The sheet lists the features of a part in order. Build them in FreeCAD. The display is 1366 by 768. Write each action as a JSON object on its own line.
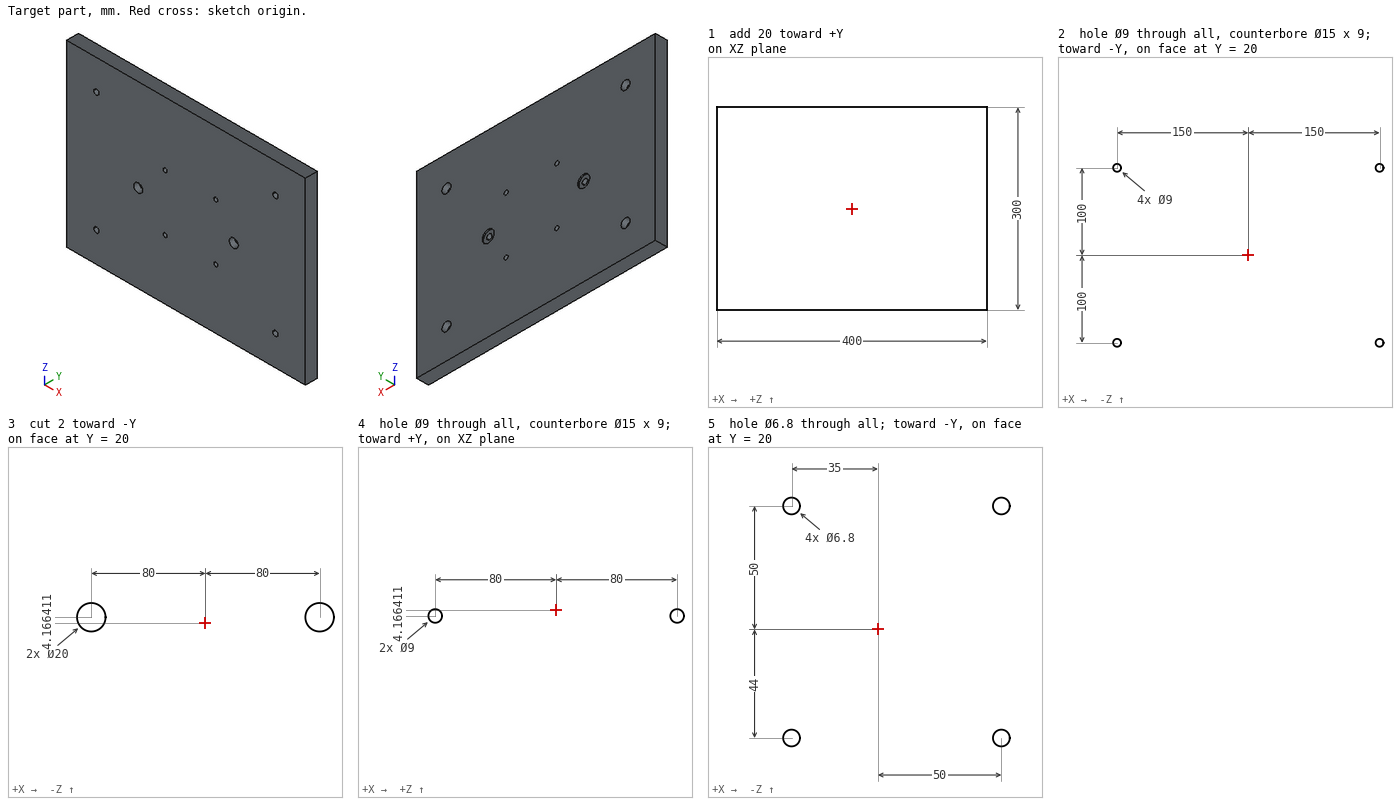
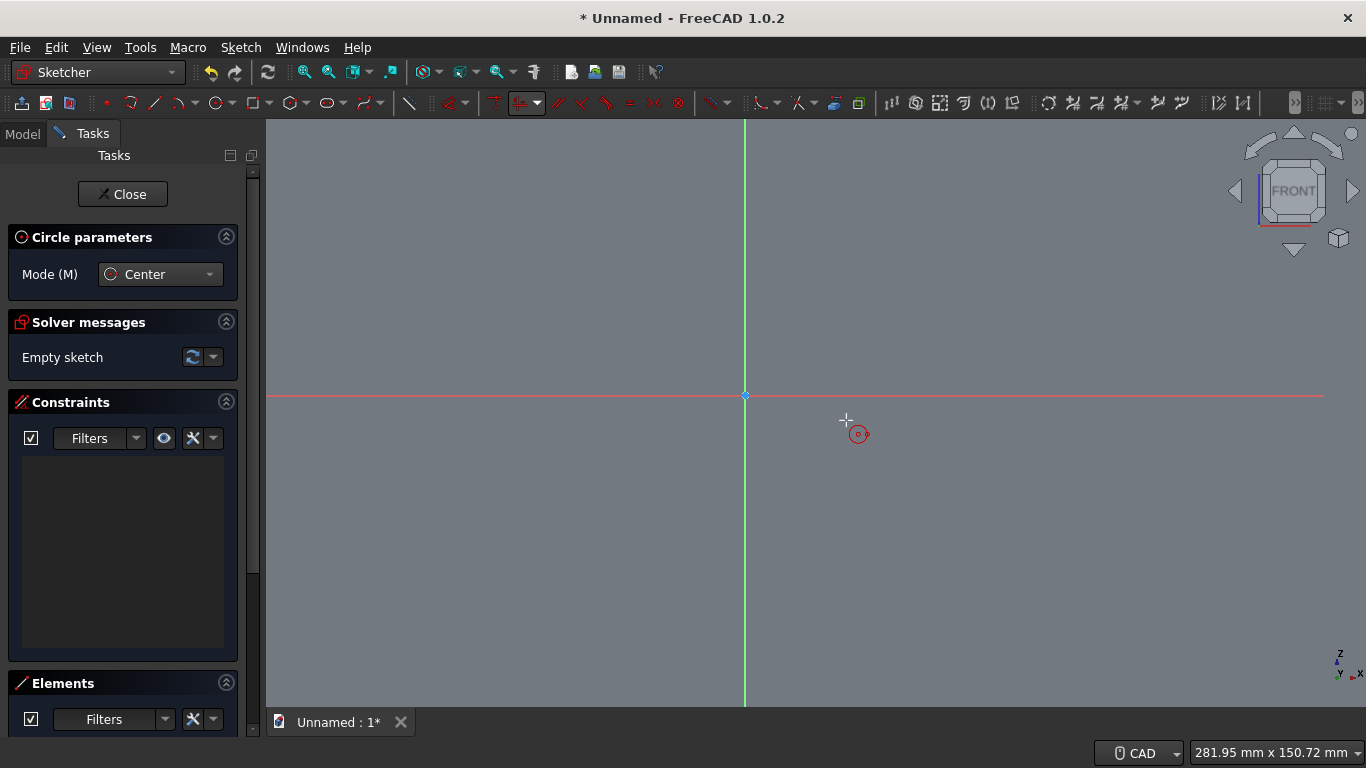
{"action": "scroll", "coordinate": [433, 412], "scroll_direction": "up", "scroll_amount": 2}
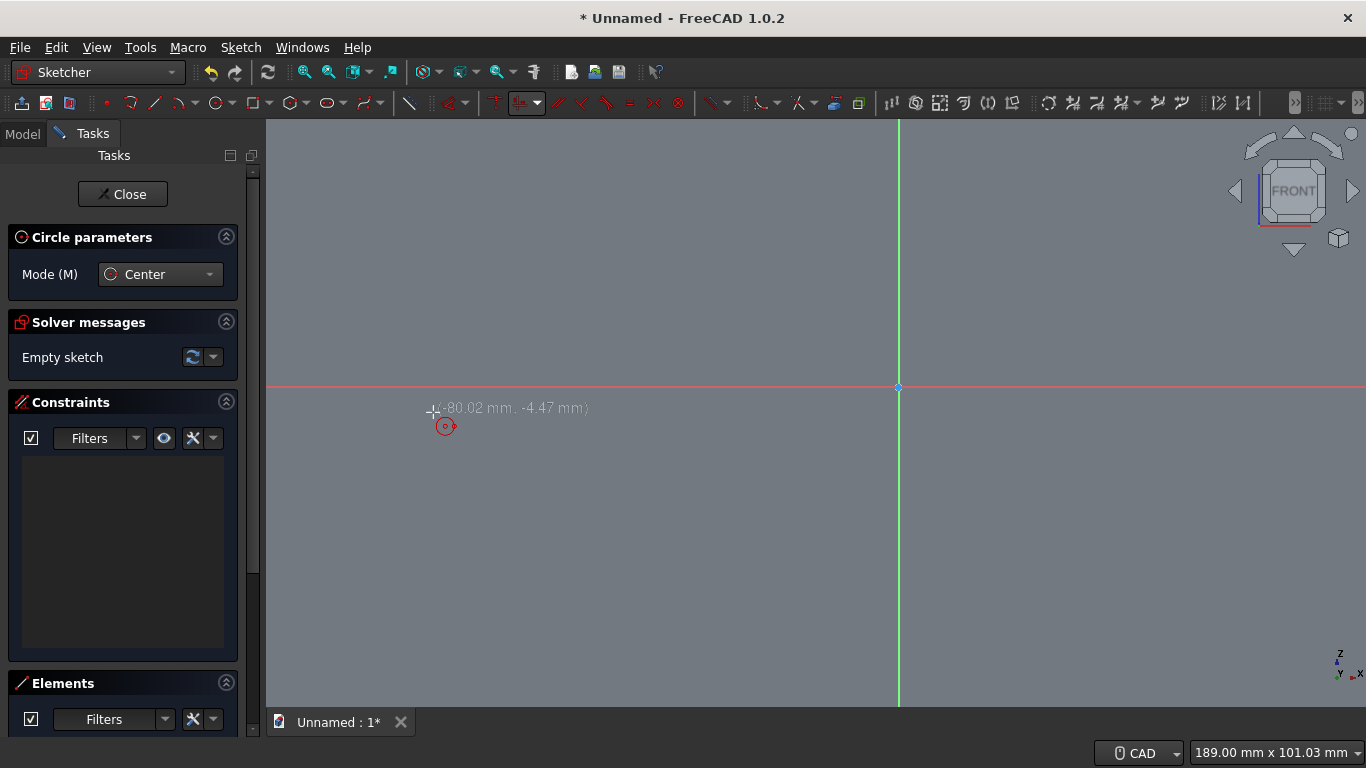
{"action": "left_click", "coordinate": [433, 411]}
{"action": "left_click", "coordinate": [452, 430]}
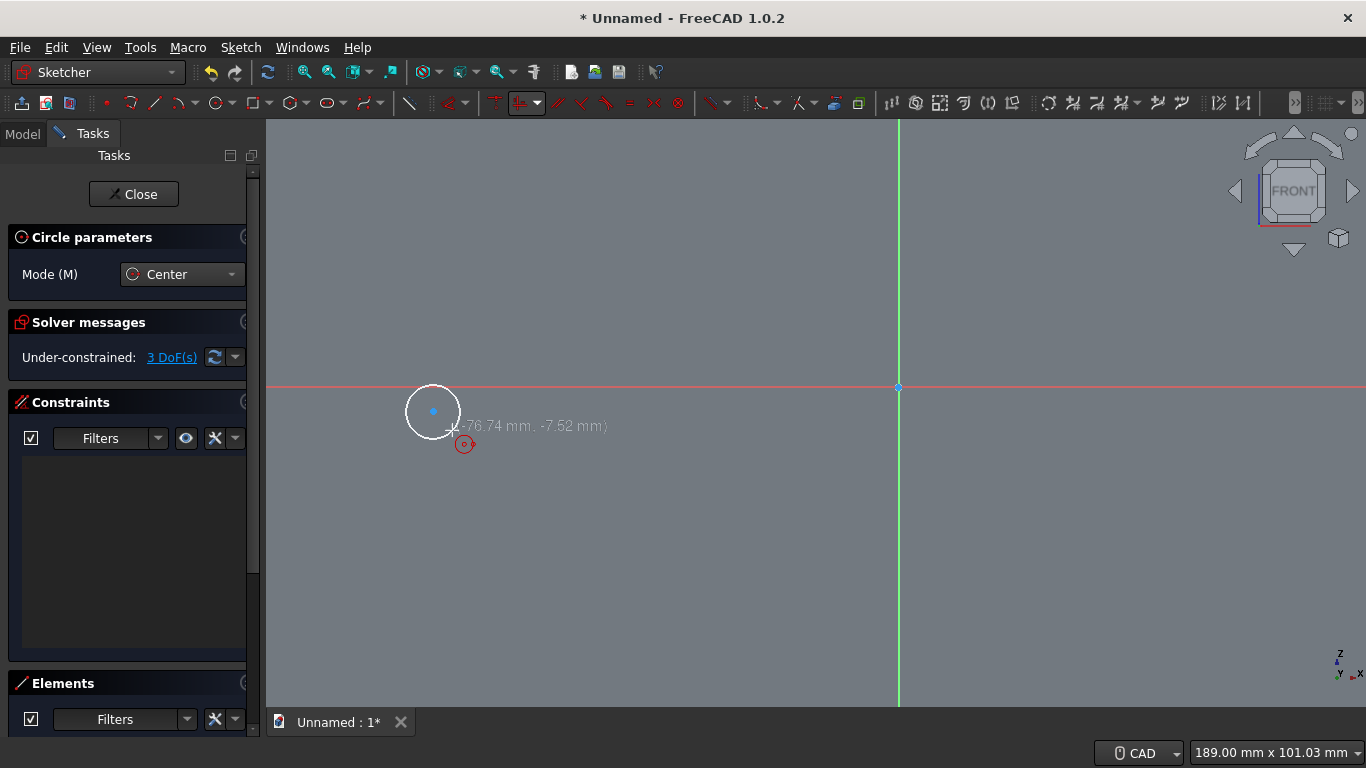
{"action": "scroll", "coordinate": [440, 416], "scroll_direction": "down", "scroll_amount": 2}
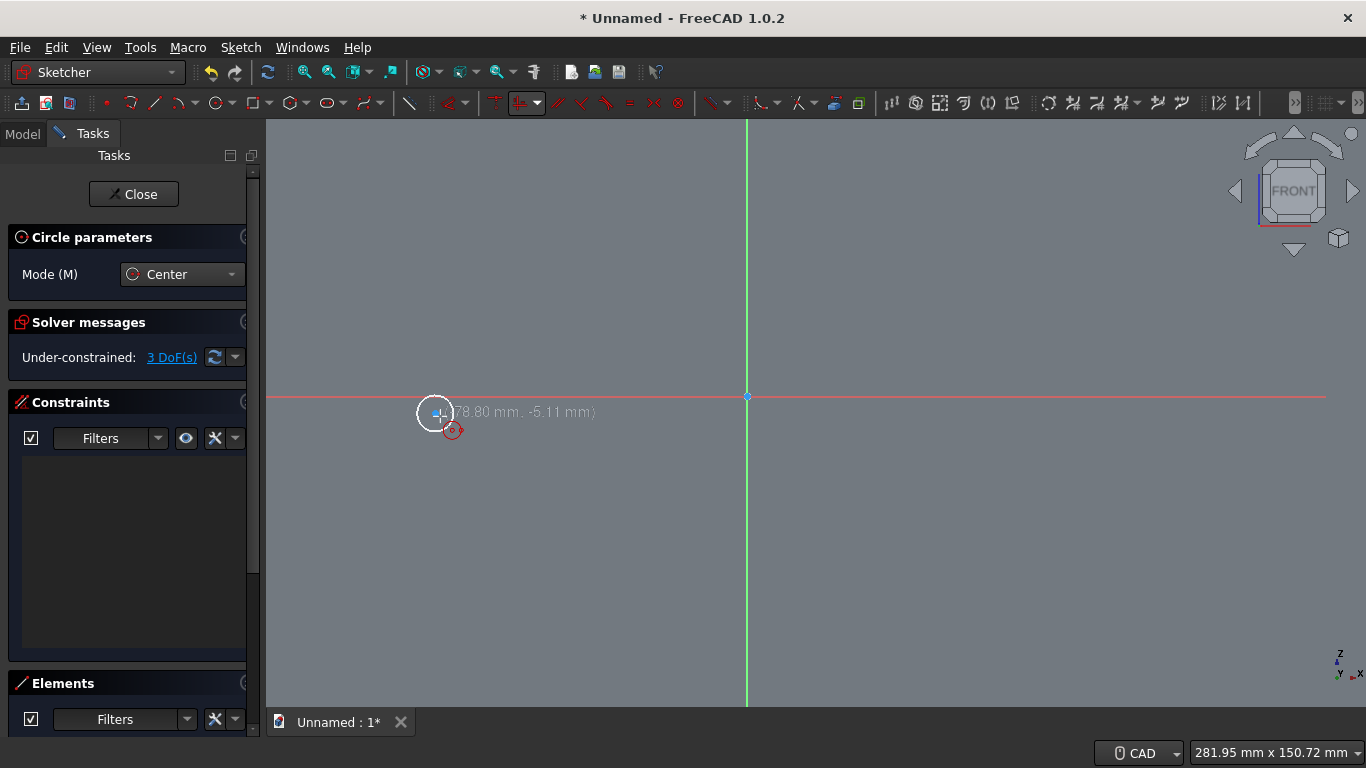
{"action": "scroll", "coordinate": [1060, 413], "scroll_direction": "up", "scroll_amount": 2}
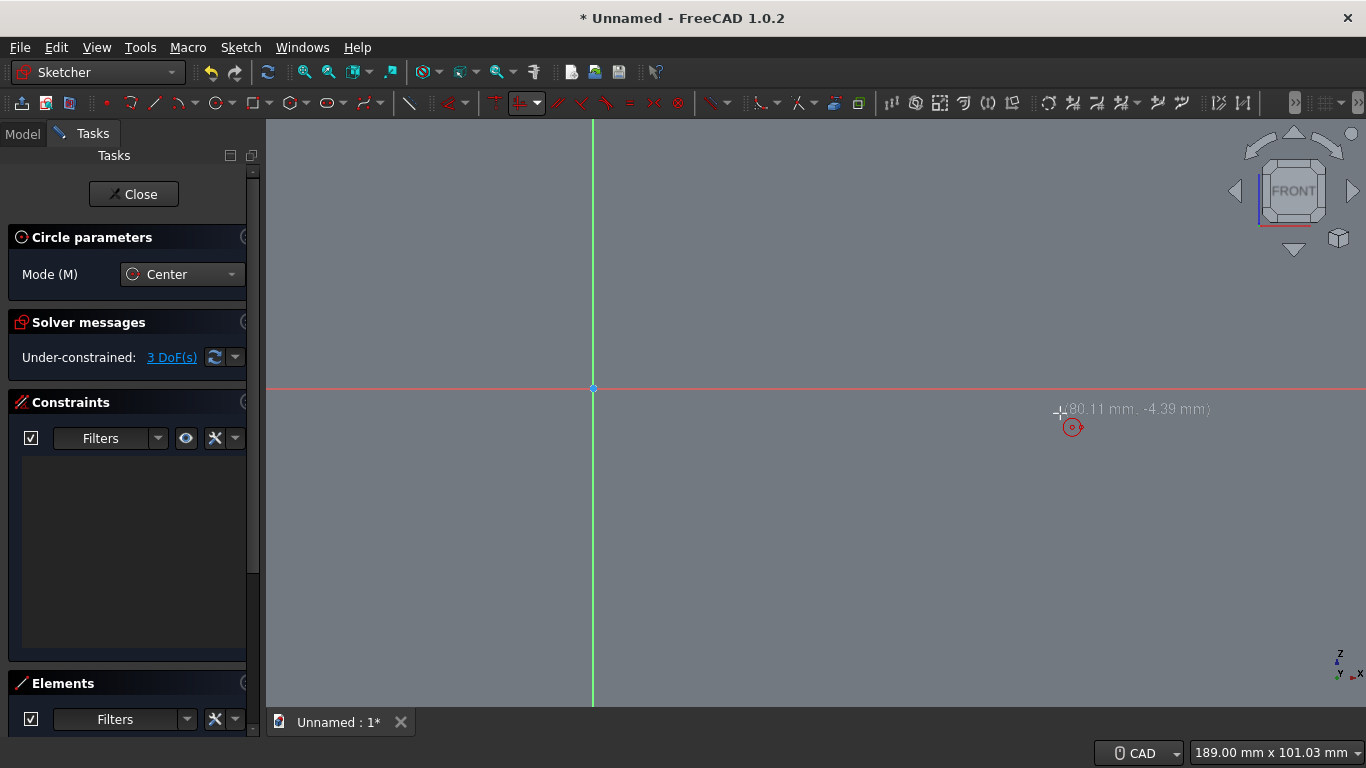
{"action": "left_click", "coordinate": [1059, 413]}
{"action": "left_click", "coordinate": [1078, 431]}
{"action": "key", "text": "Escape"}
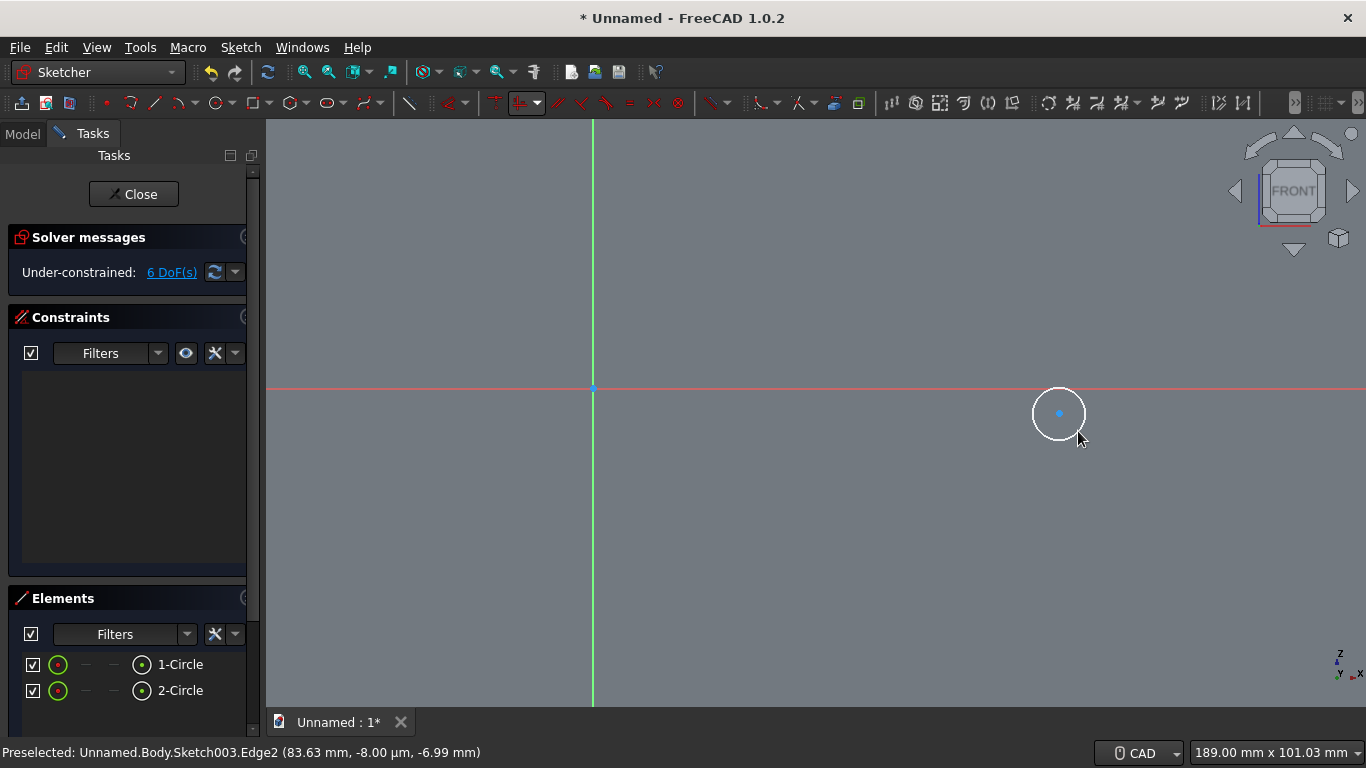
{"action": "scroll", "coordinate": [1061, 413], "scroll_direction": "down", "scroll_amount": 2}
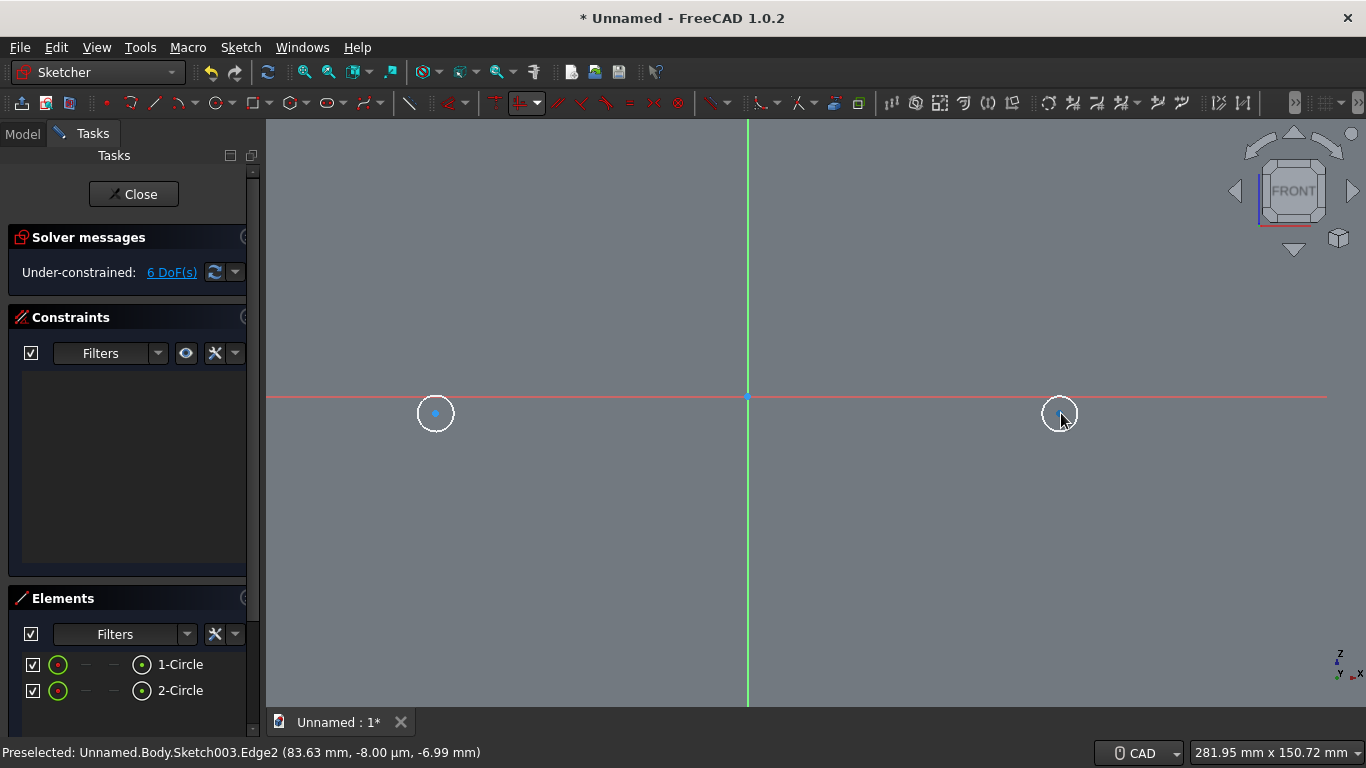
{"action": "left_click", "coordinate": [423, 426]}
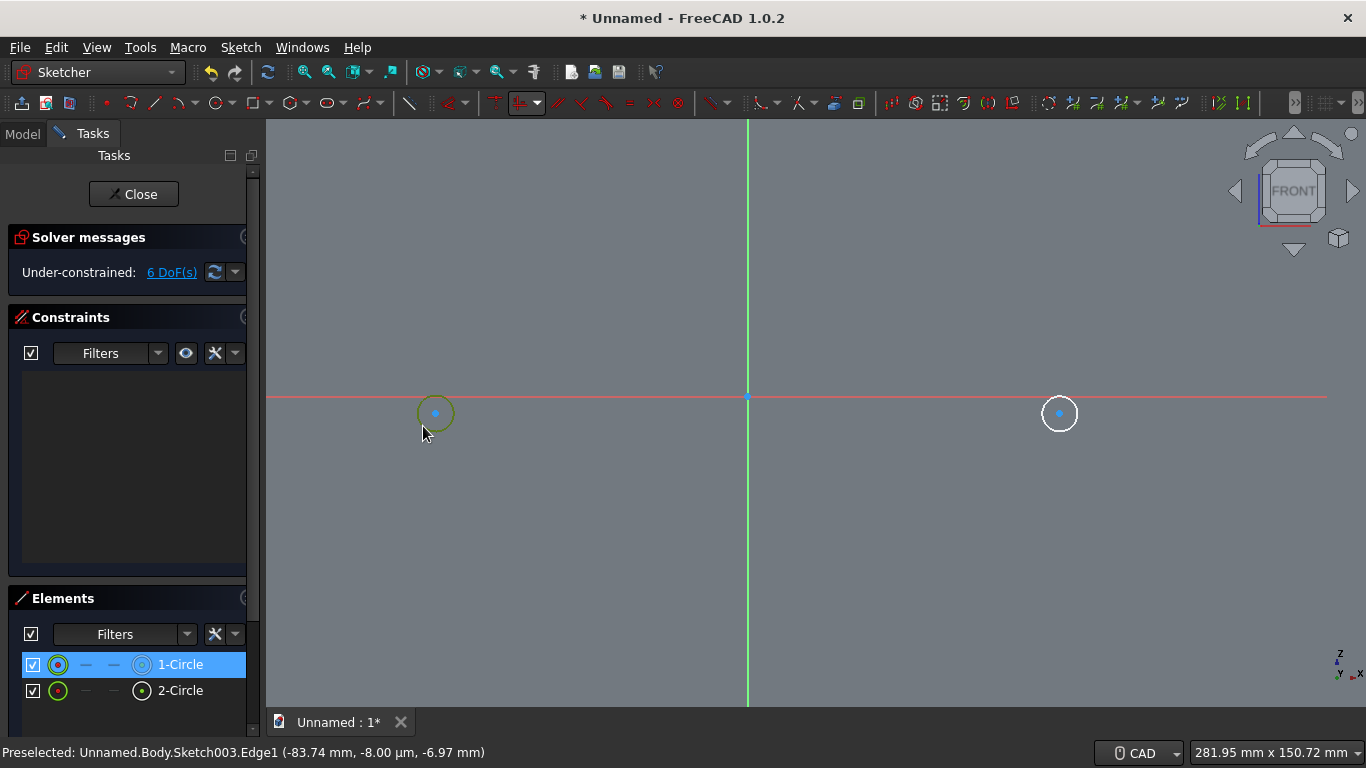
{"action": "left_click", "coordinate": [1048, 426]}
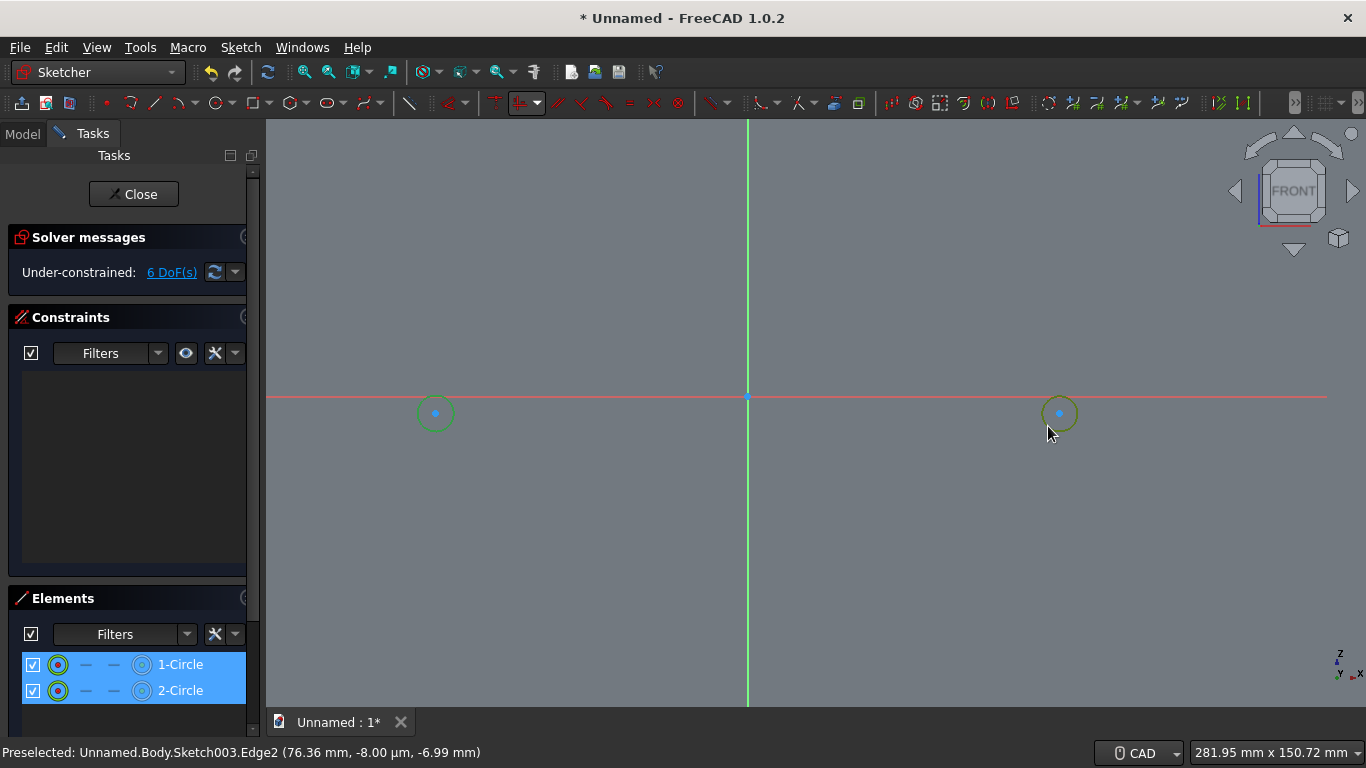
{"action": "key", "text": "e"}